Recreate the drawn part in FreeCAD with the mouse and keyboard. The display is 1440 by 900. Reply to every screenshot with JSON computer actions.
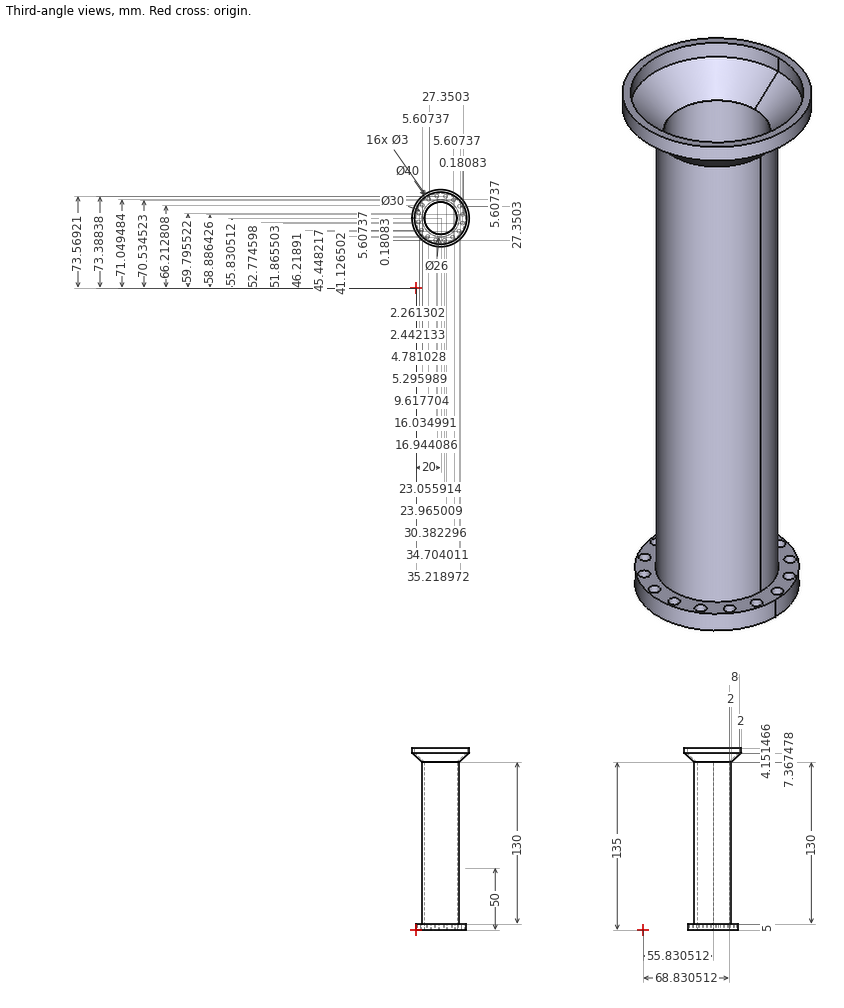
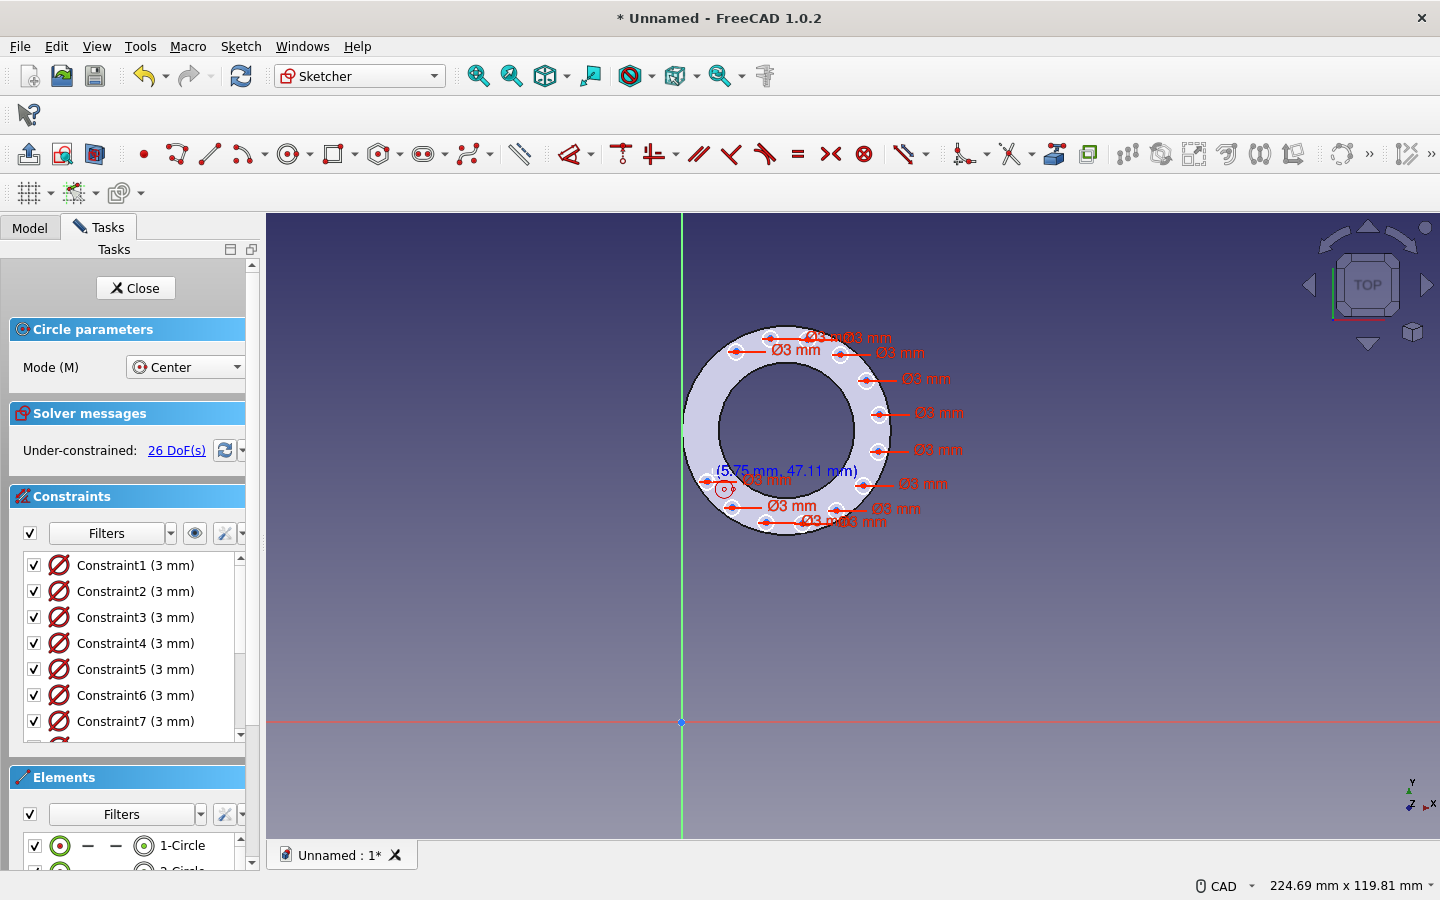
{"action": "scroll", "coordinate": [694, 446], "scroll_direction": "up", "scroll_amount": 6}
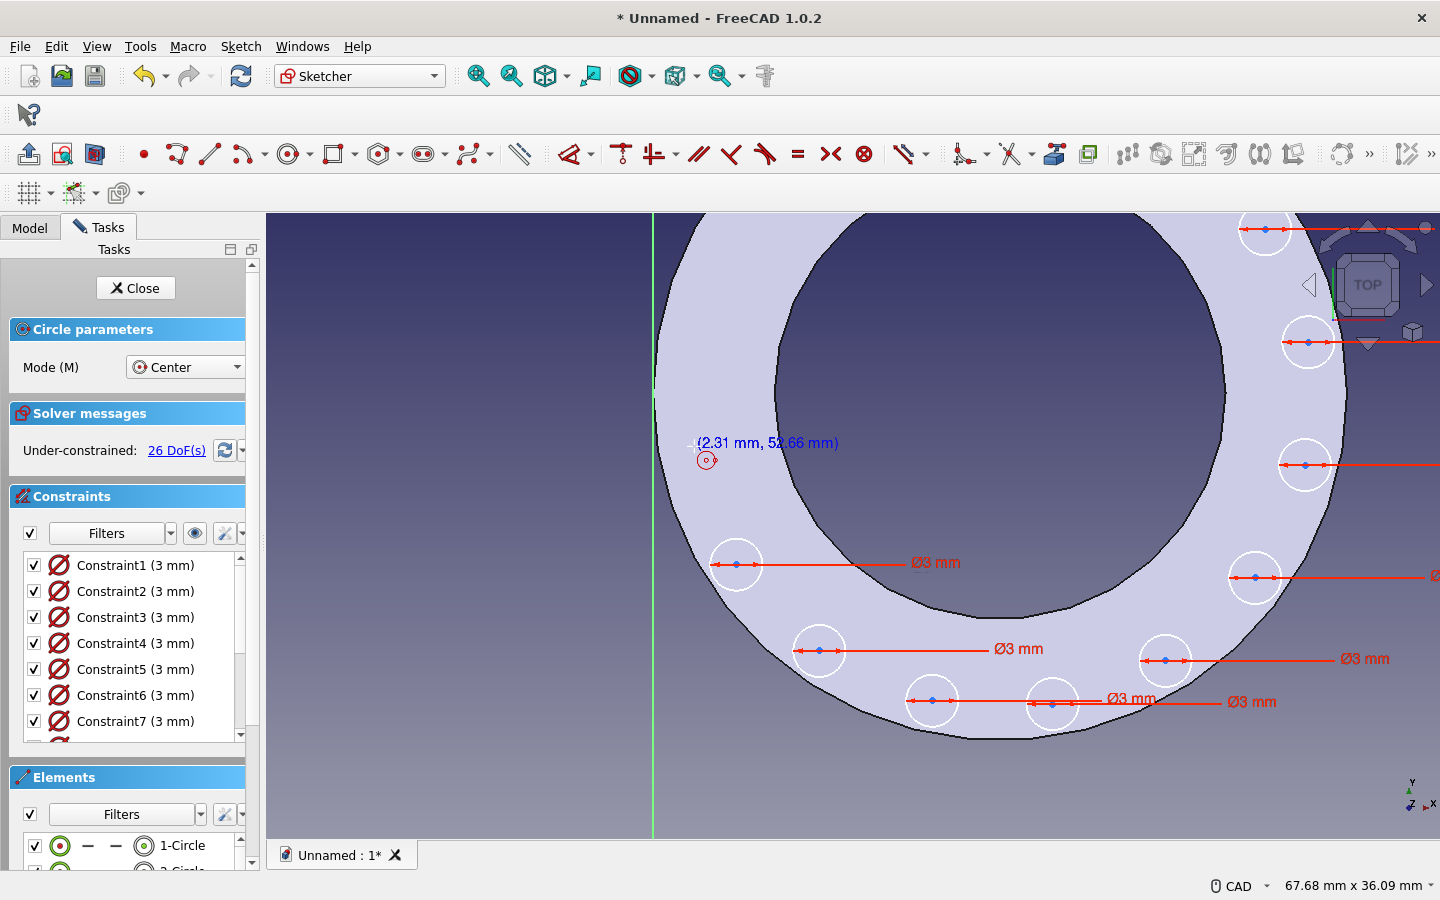
{"action": "left_click", "coordinate": [692, 446]}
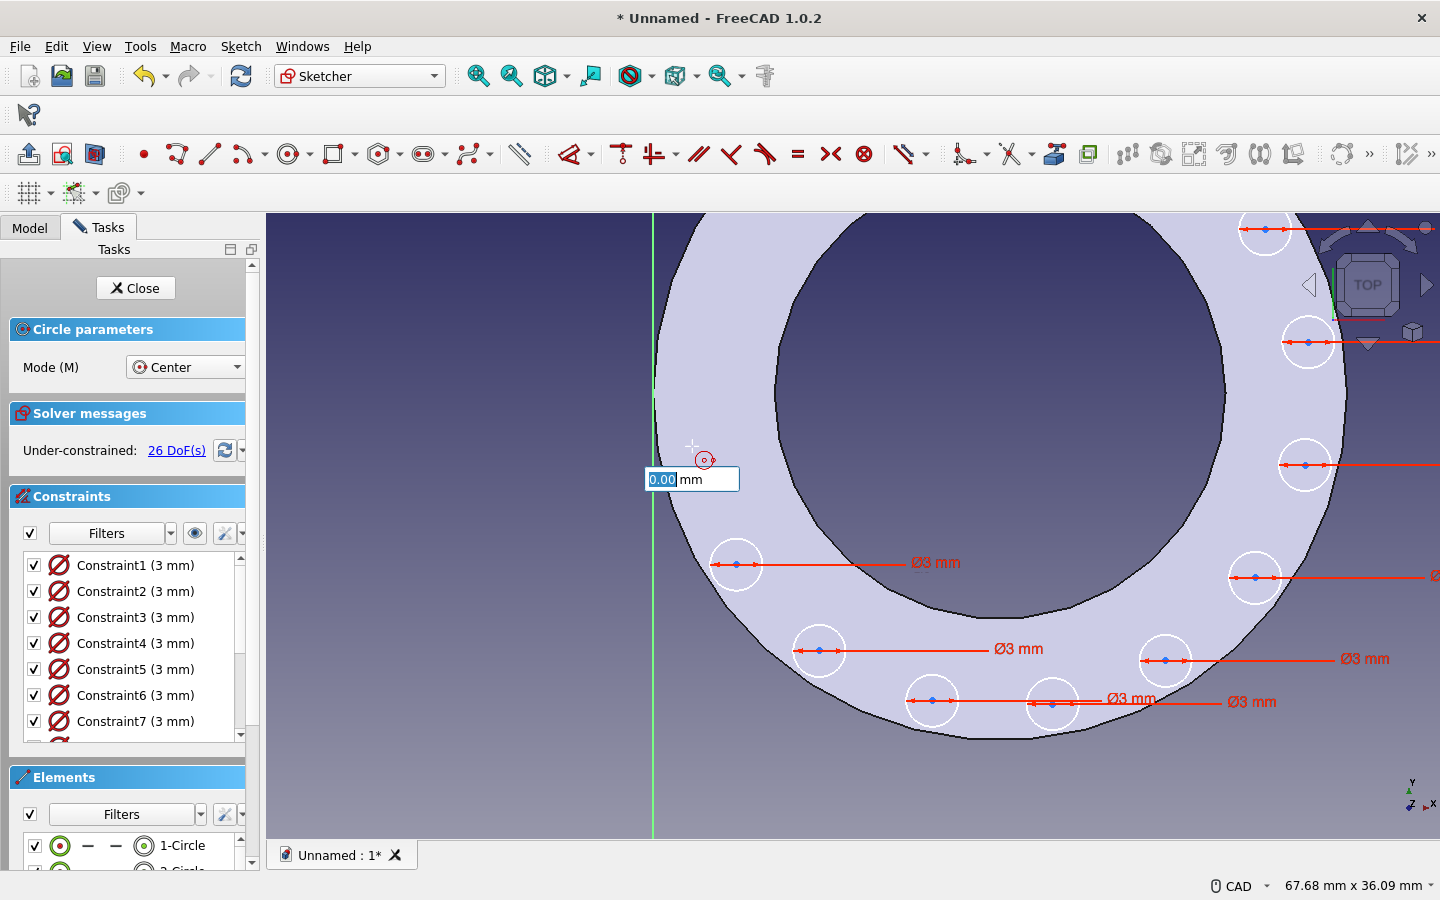
{"action": "scroll", "coordinate": [694, 446], "scroll_direction": "down", "scroll_amount": 6}
{"action": "mouse_move", "coordinate": [699, 441]}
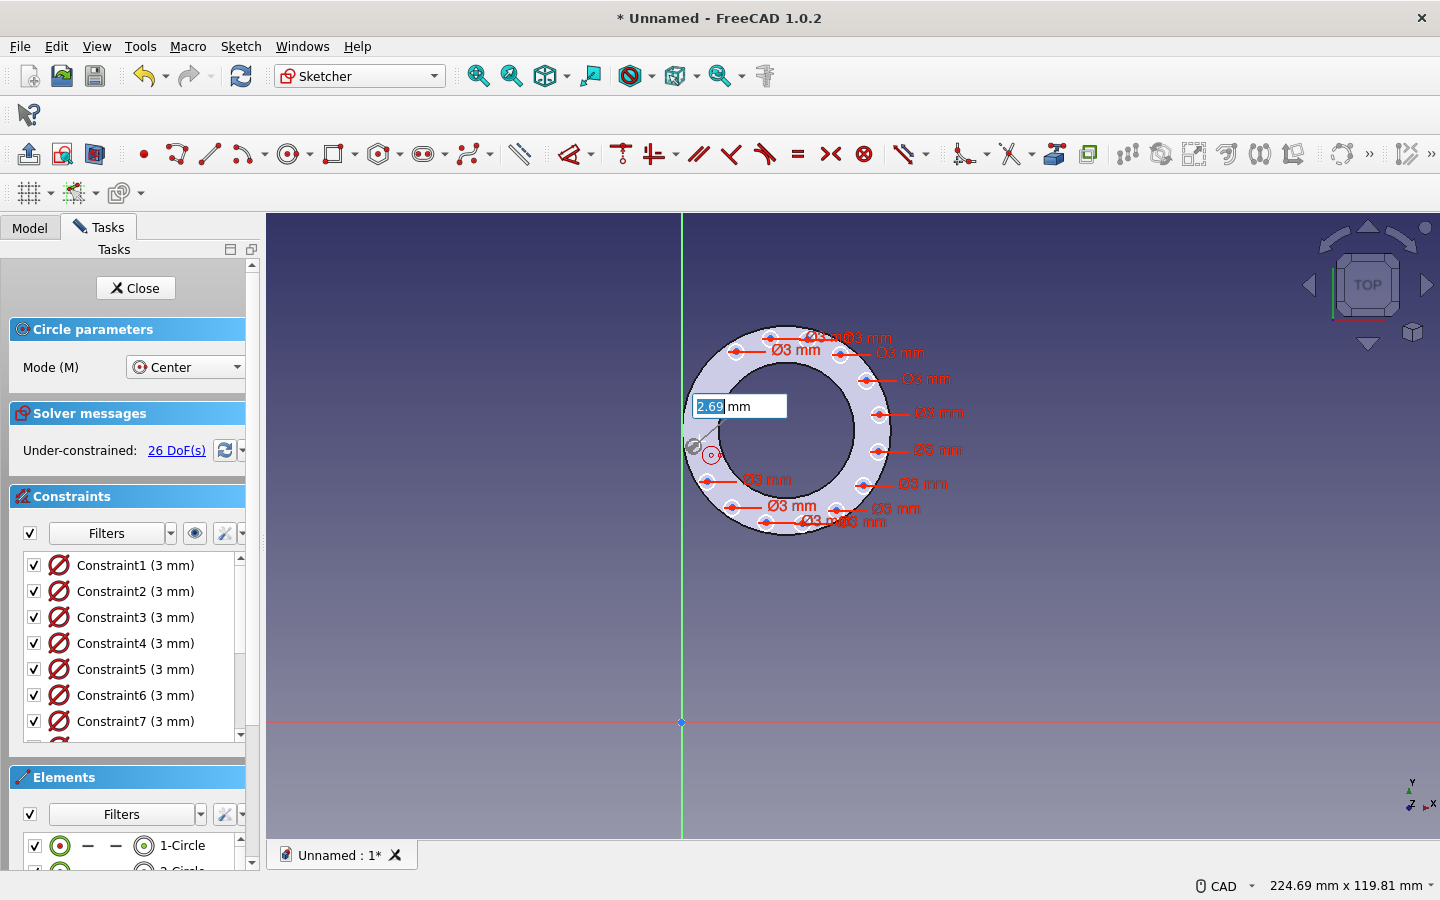
{"action": "type", "text": "3"}
{"action": "key", "text": "Return"}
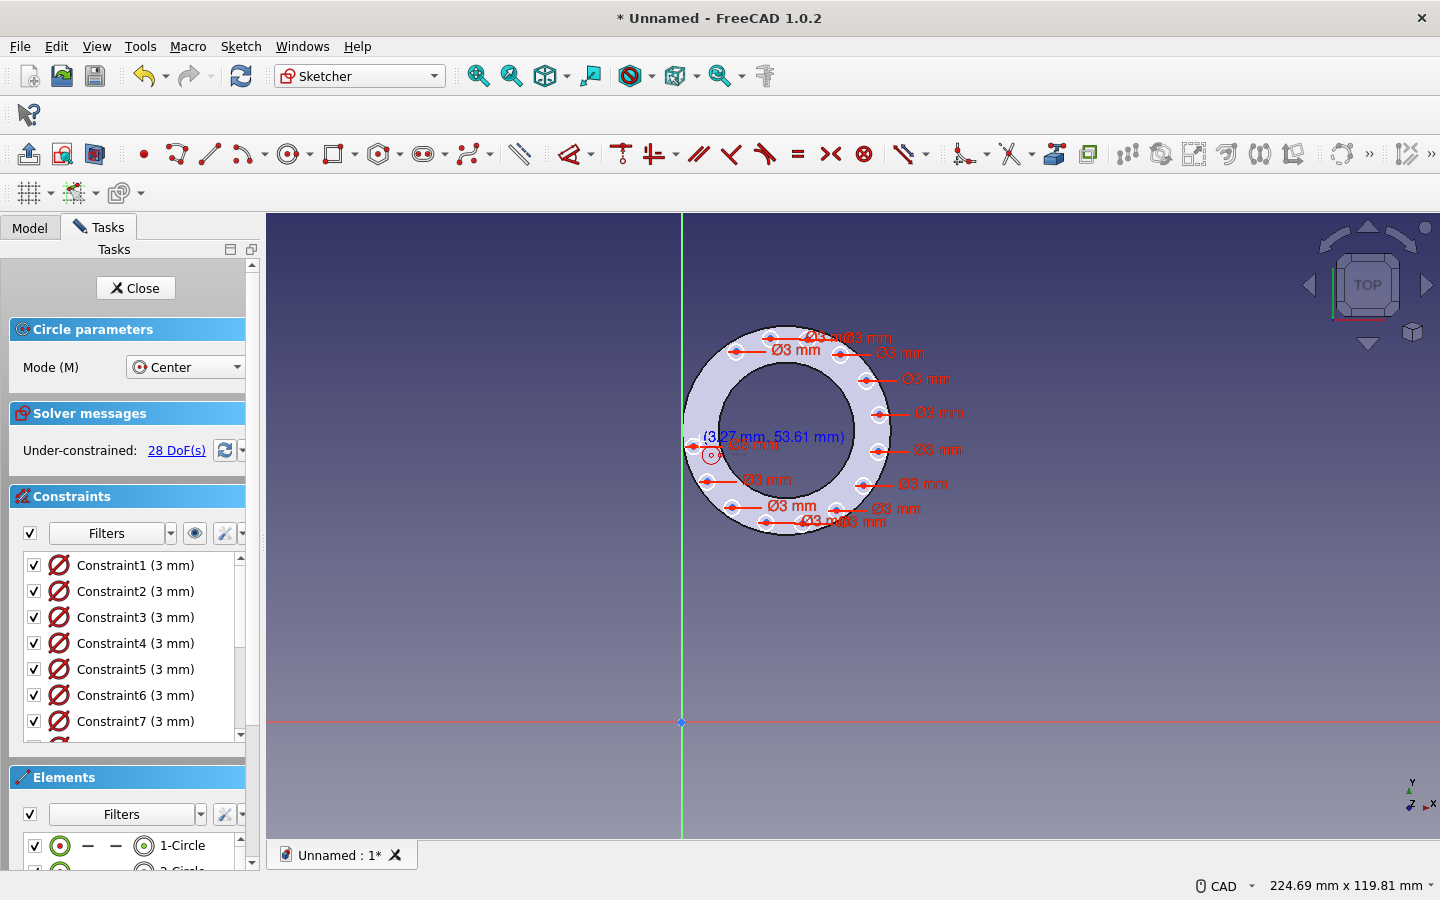
{"action": "scroll", "coordinate": [695, 410], "scroll_direction": "up", "scroll_amount": 6}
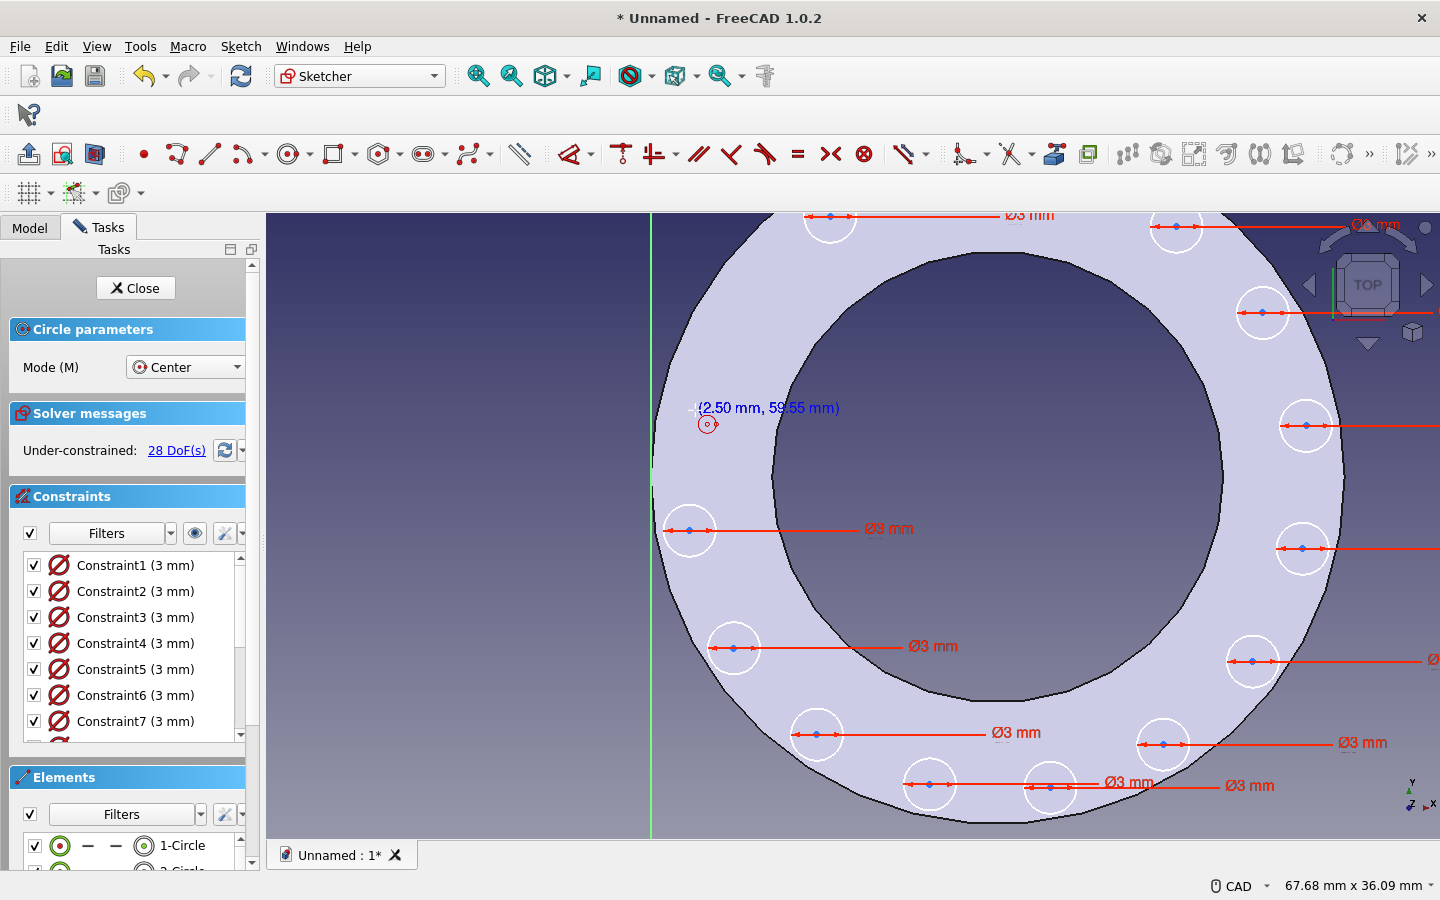
{"action": "left_click", "coordinate": [693, 408]}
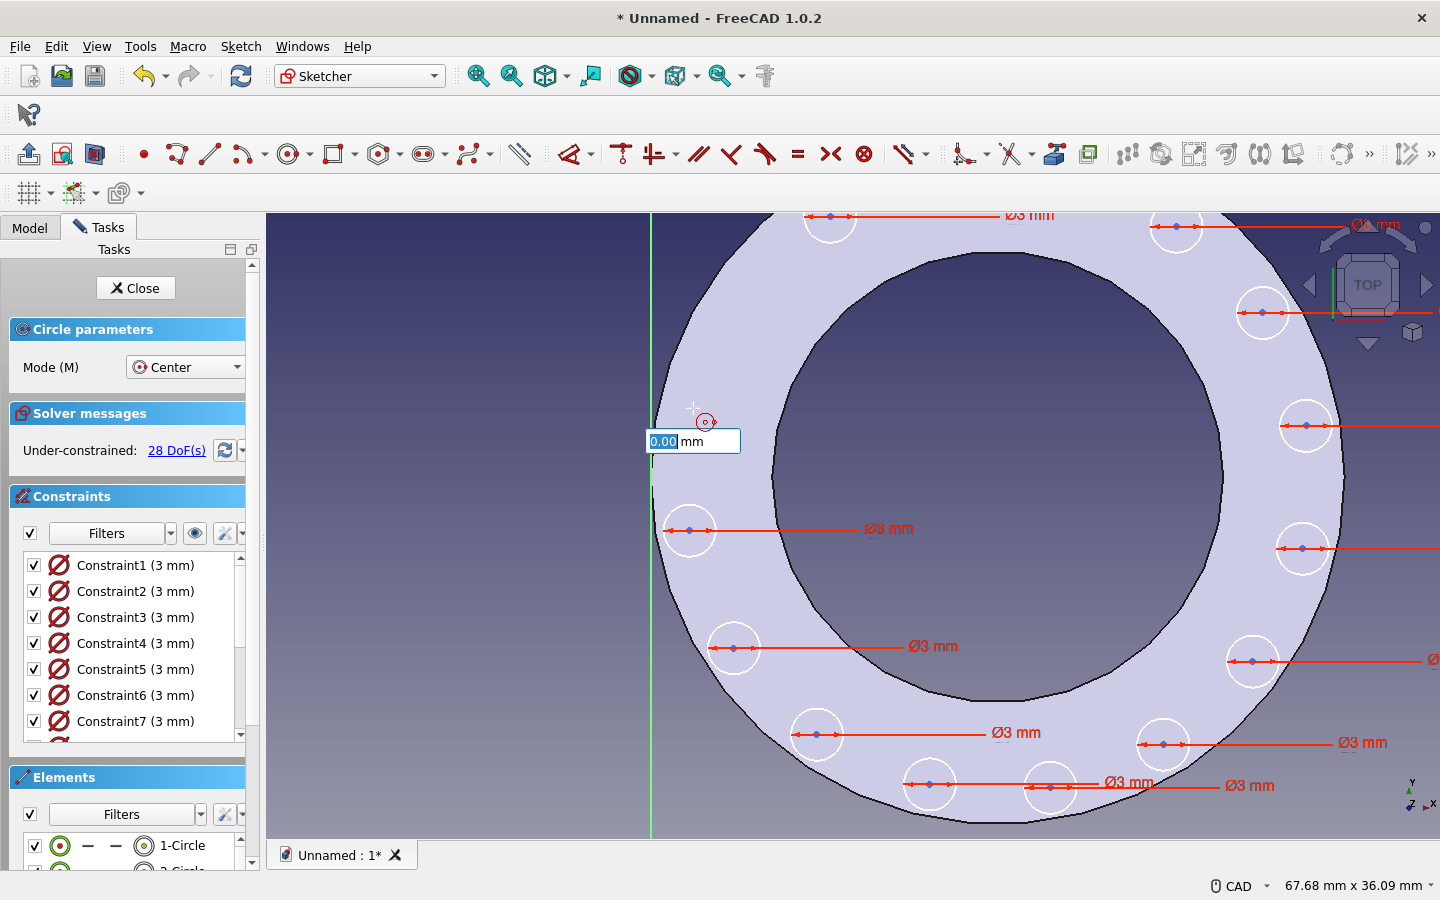
{"action": "scroll", "coordinate": [695, 410], "scroll_direction": "down", "scroll_amount": 6}
{"action": "mouse_move", "coordinate": [700, 404]}